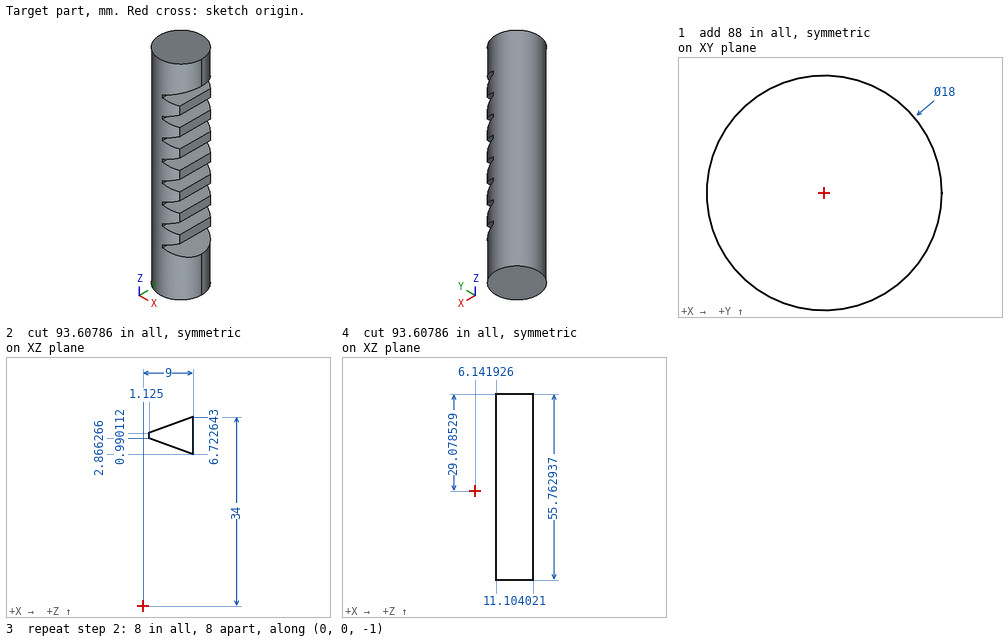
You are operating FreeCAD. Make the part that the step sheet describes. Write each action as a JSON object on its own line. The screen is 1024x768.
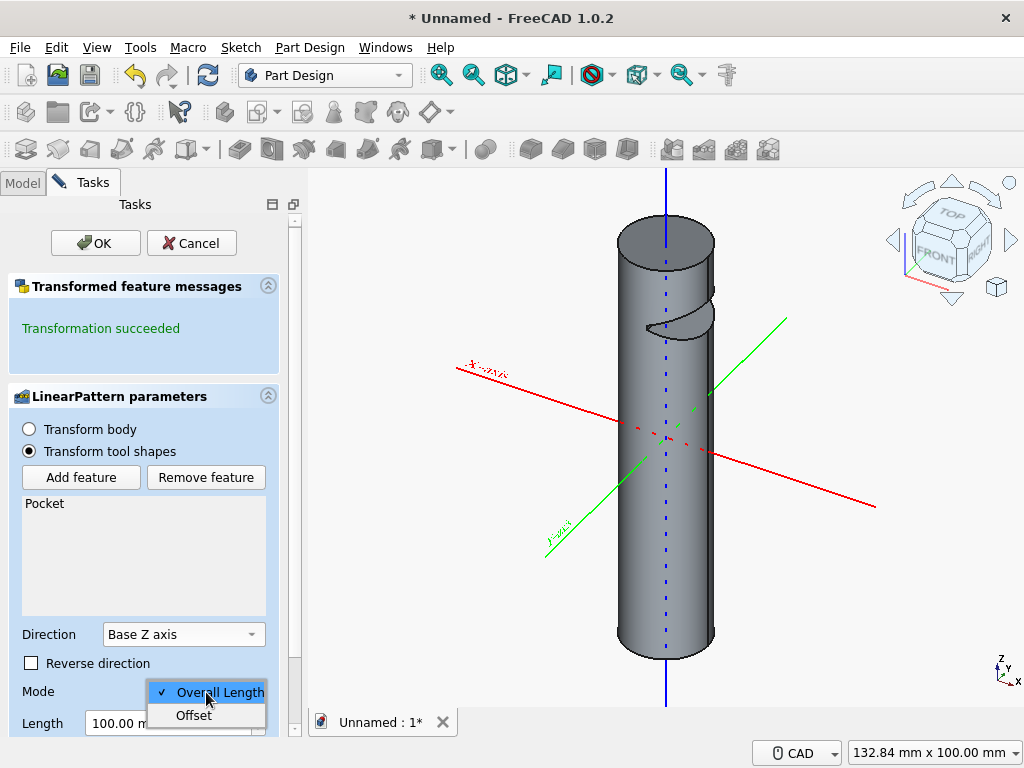
{"action": "left_click", "coordinate": [206, 716]}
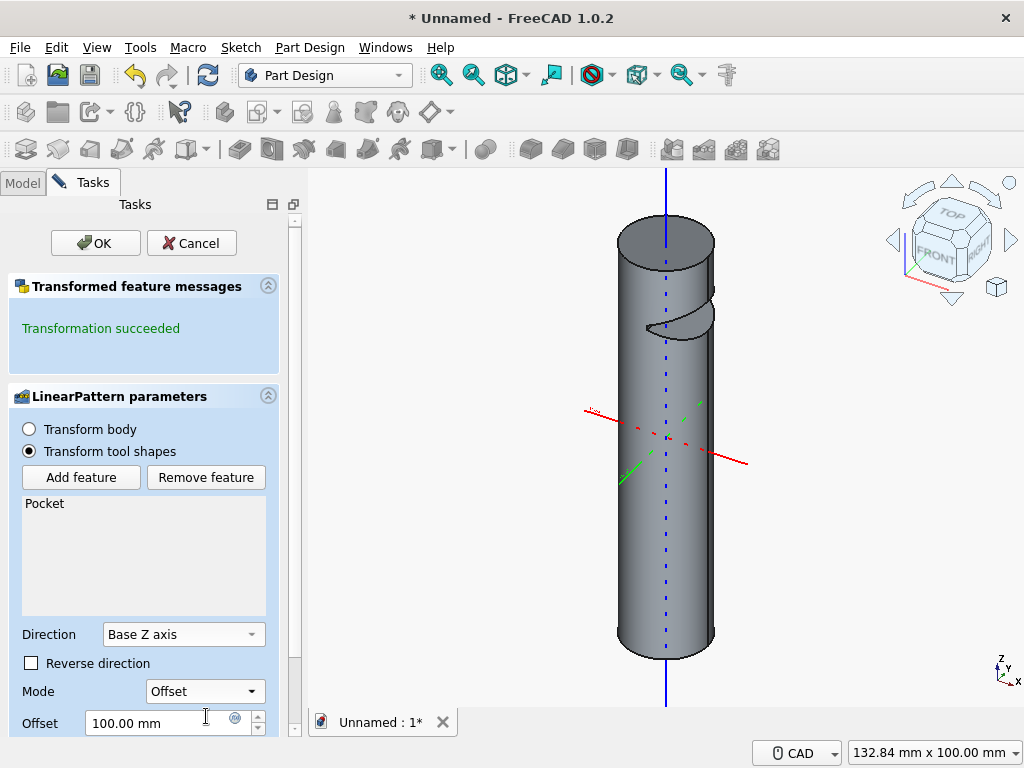
{"action": "triple_click", "coordinate": [168, 723]}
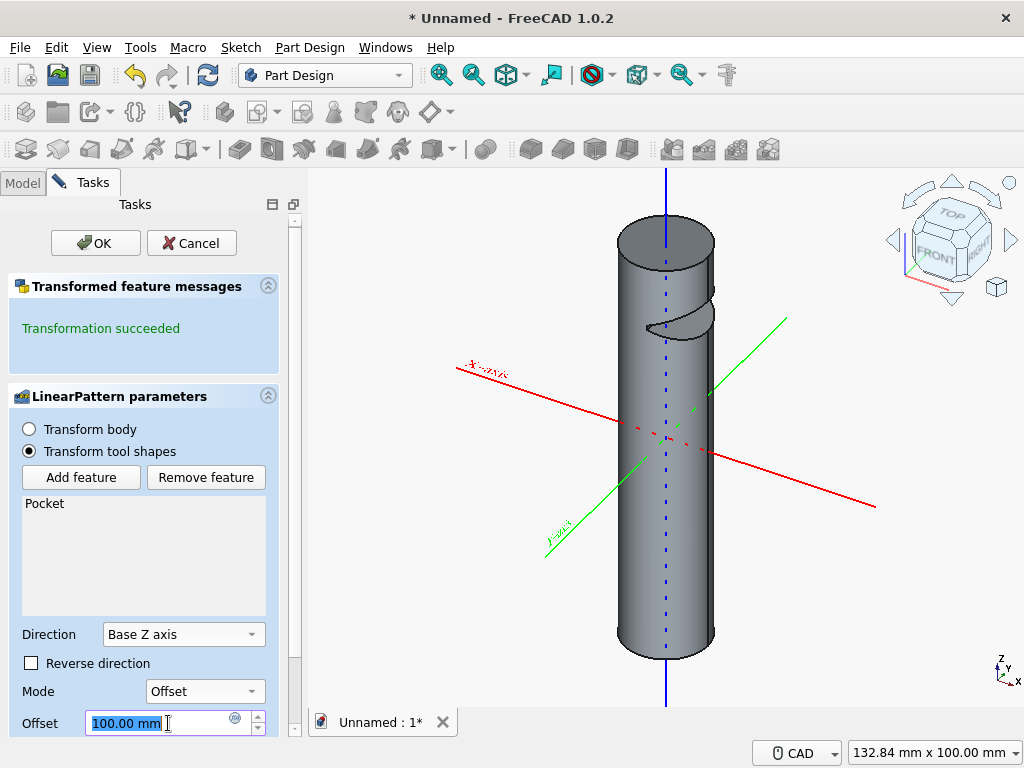
{"action": "type", "text": "8"}
{"action": "key", "text": "Tab"}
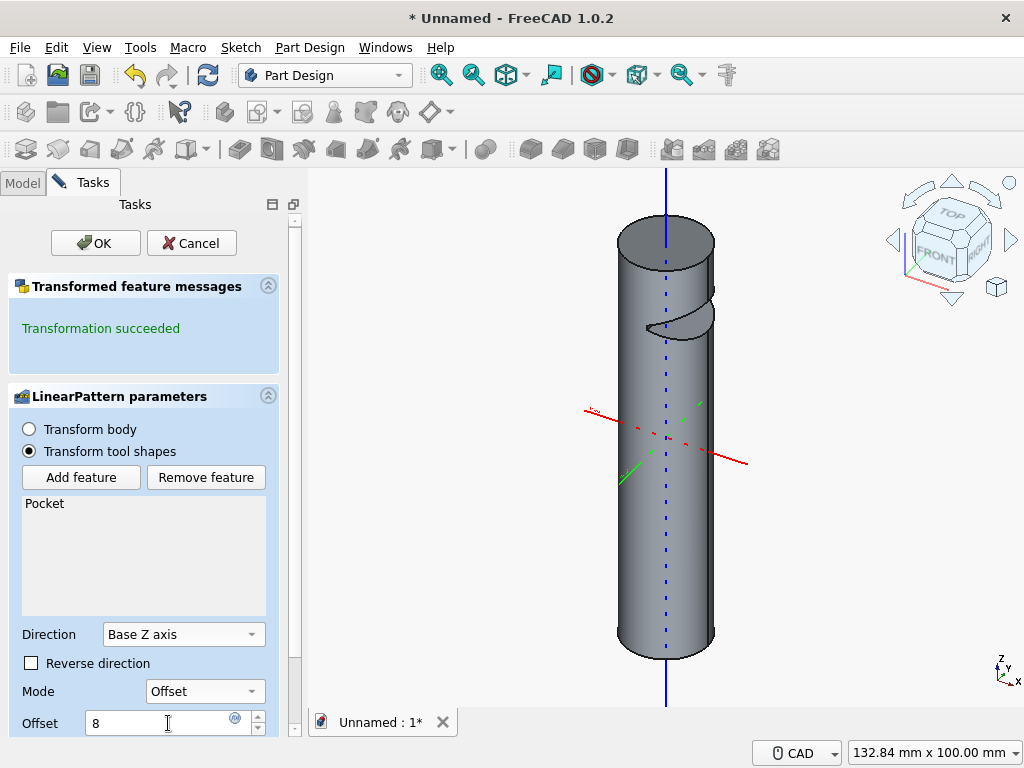
{"action": "scroll", "coordinate": [295, 475], "scroll_direction": "down", "scroll_amount": 2}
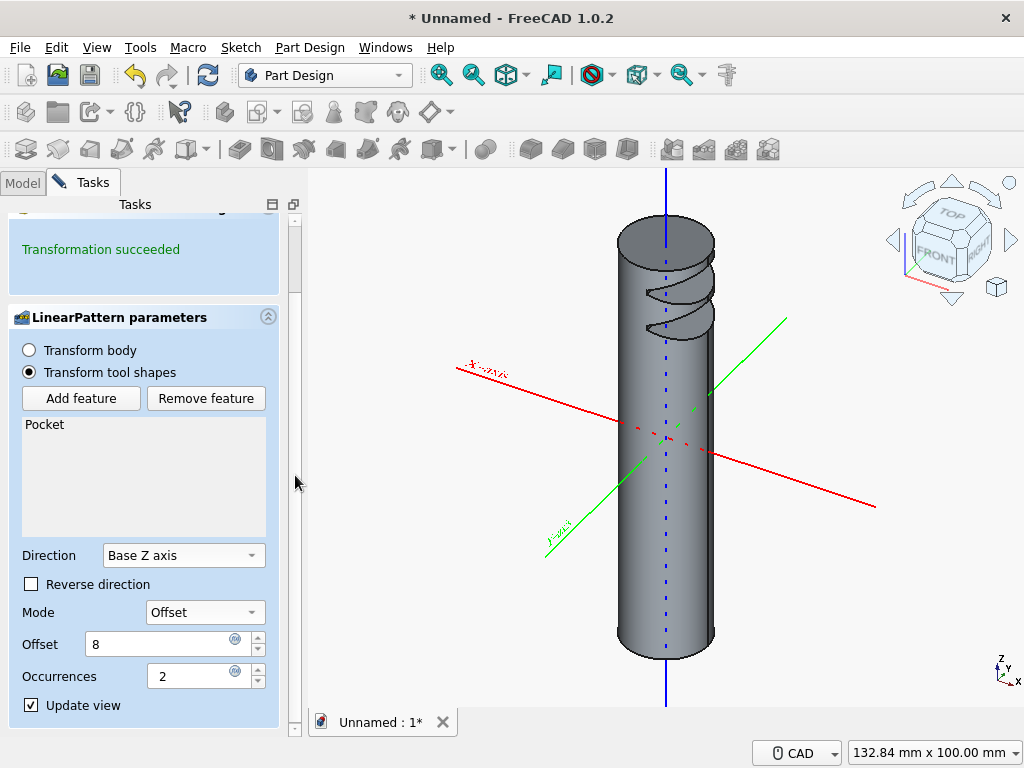
{"action": "triple_click", "coordinate": [198, 676]}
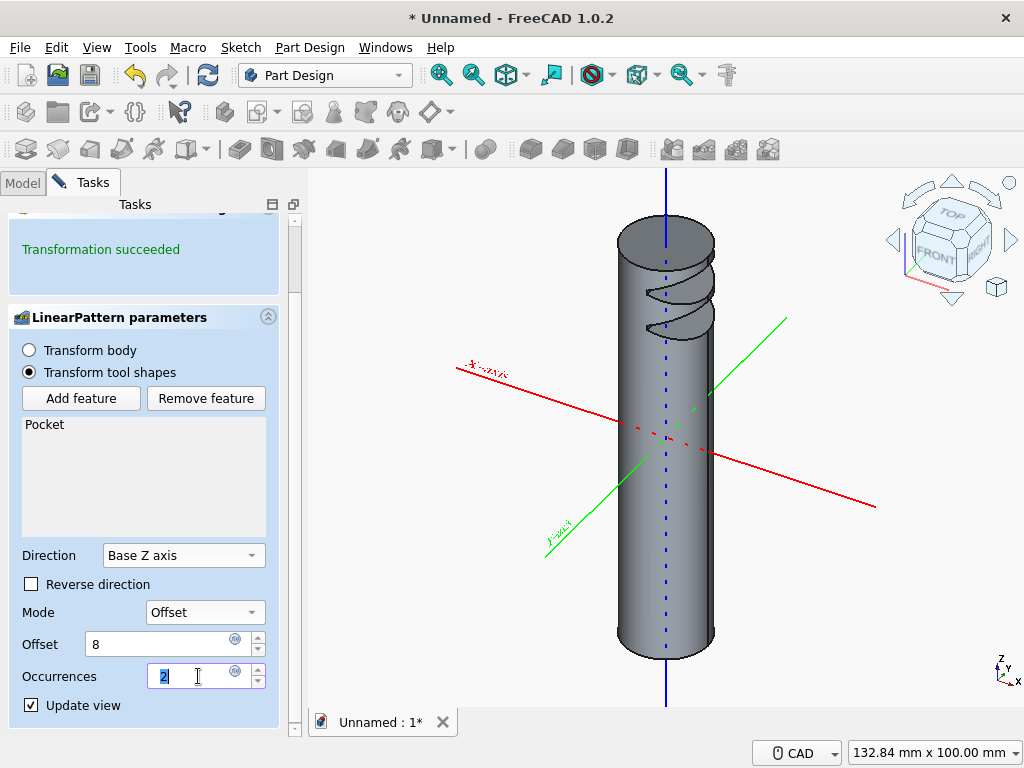
{"action": "type", "text": "8"}
{"action": "key", "text": "Tab"}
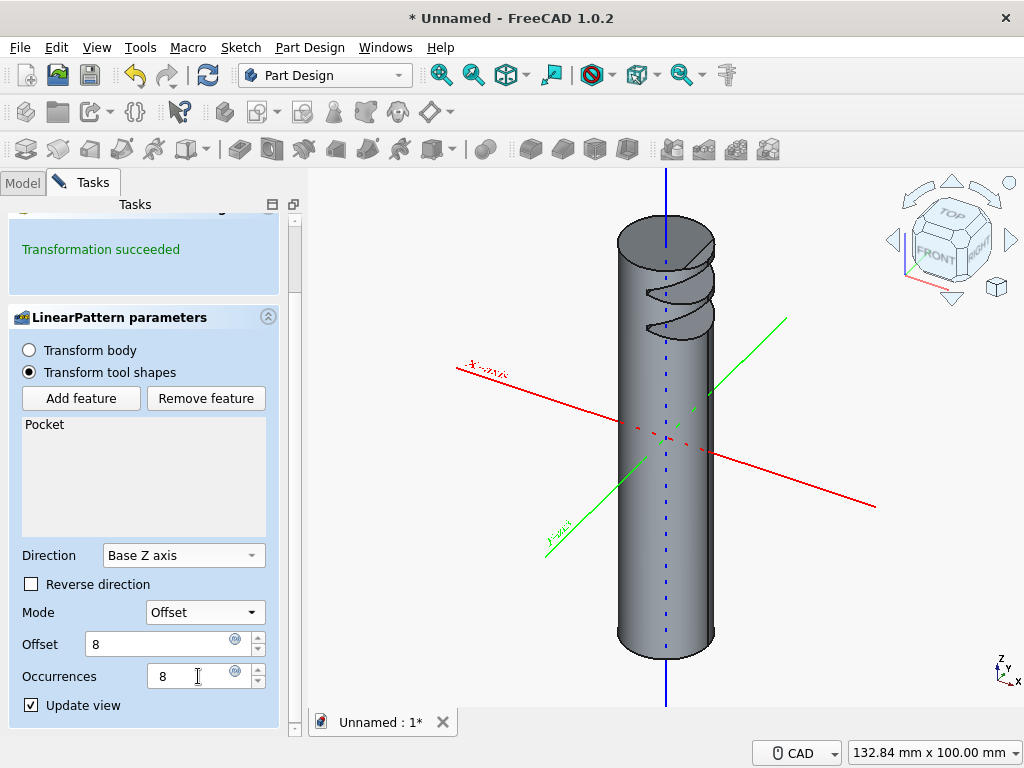
{"action": "left_click", "coordinate": [30, 584]}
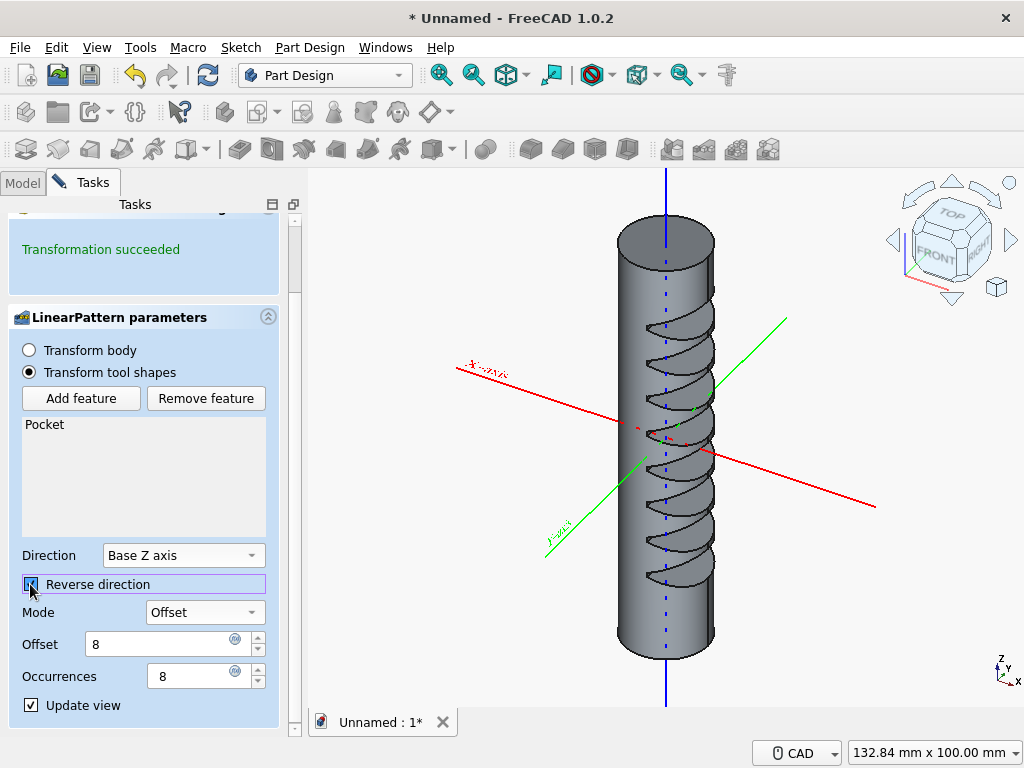
{"action": "scroll", "coordinate": [295, 475], "scroll_direction": "up", "scroll_amount": 3}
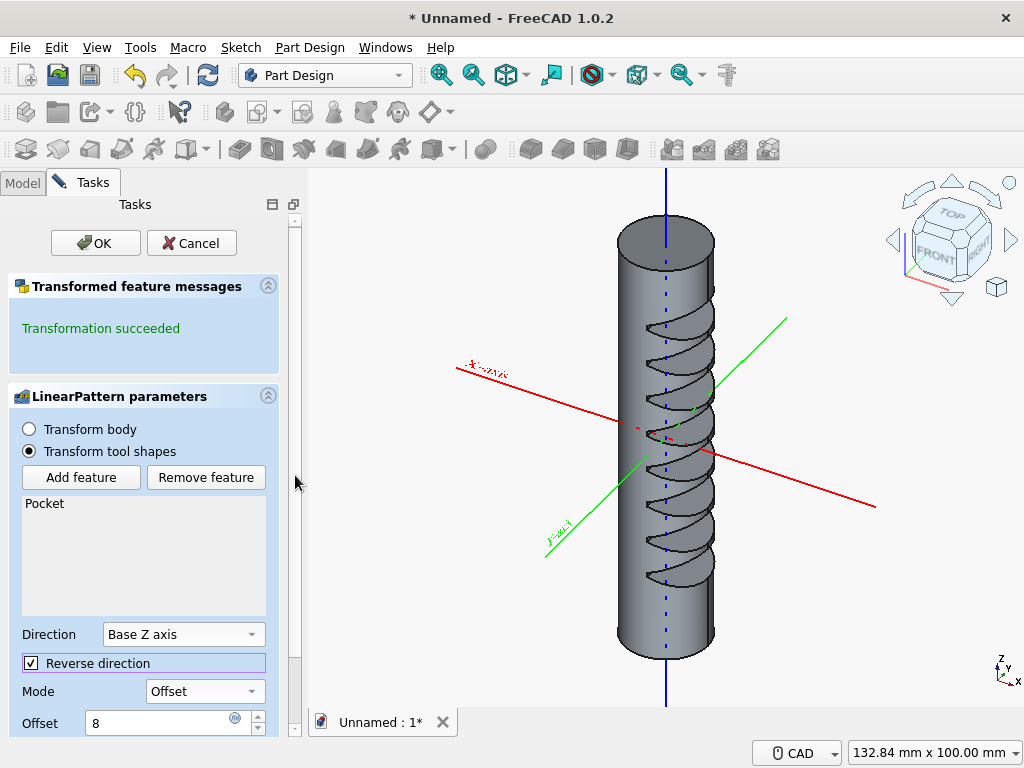
{"action": "left_click", "coordinate": [96, 243]}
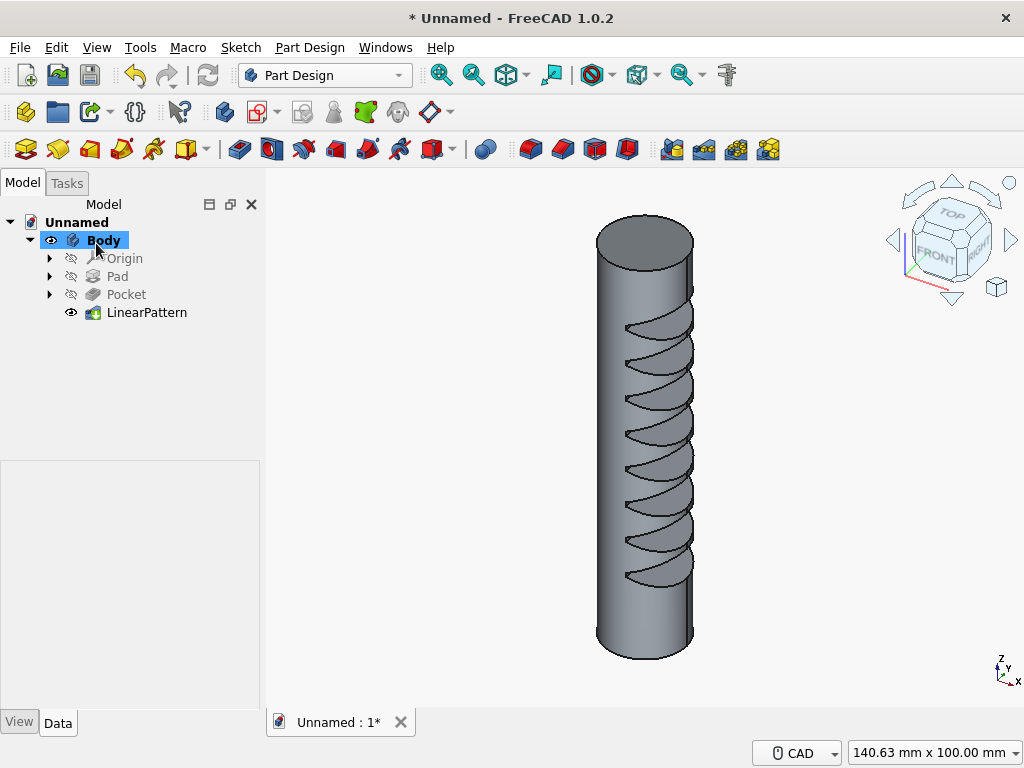
{"action": "left_click", "coordinate": [258, 112]}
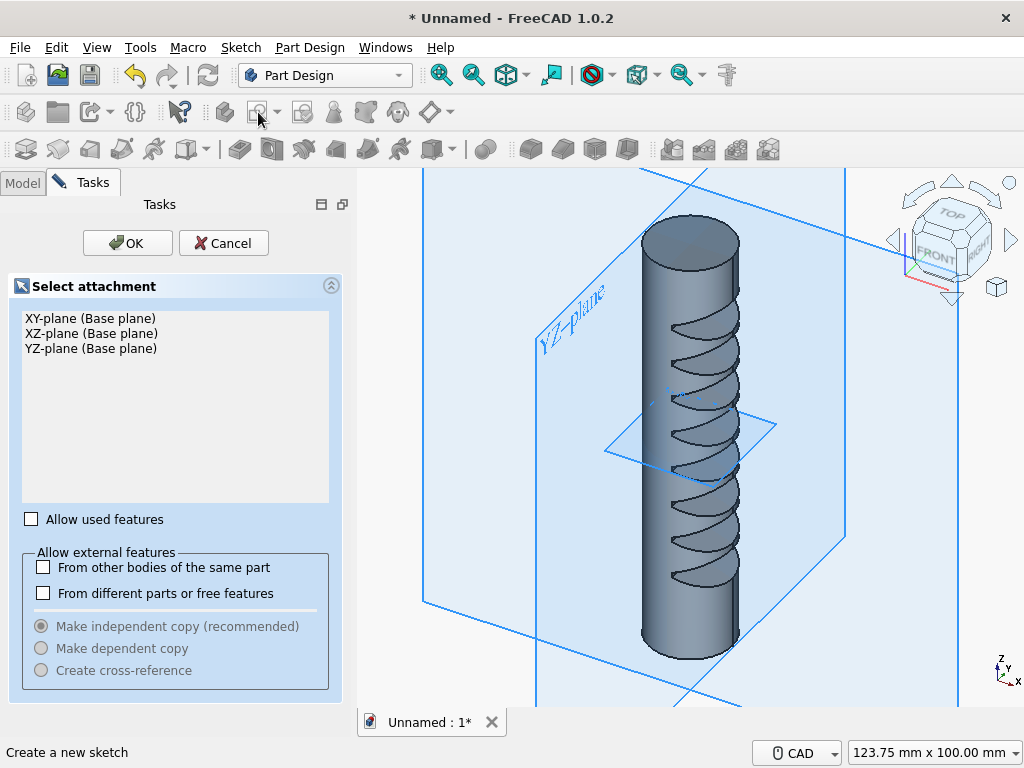
{"action": "left_click", "coordinate": [82, 334]}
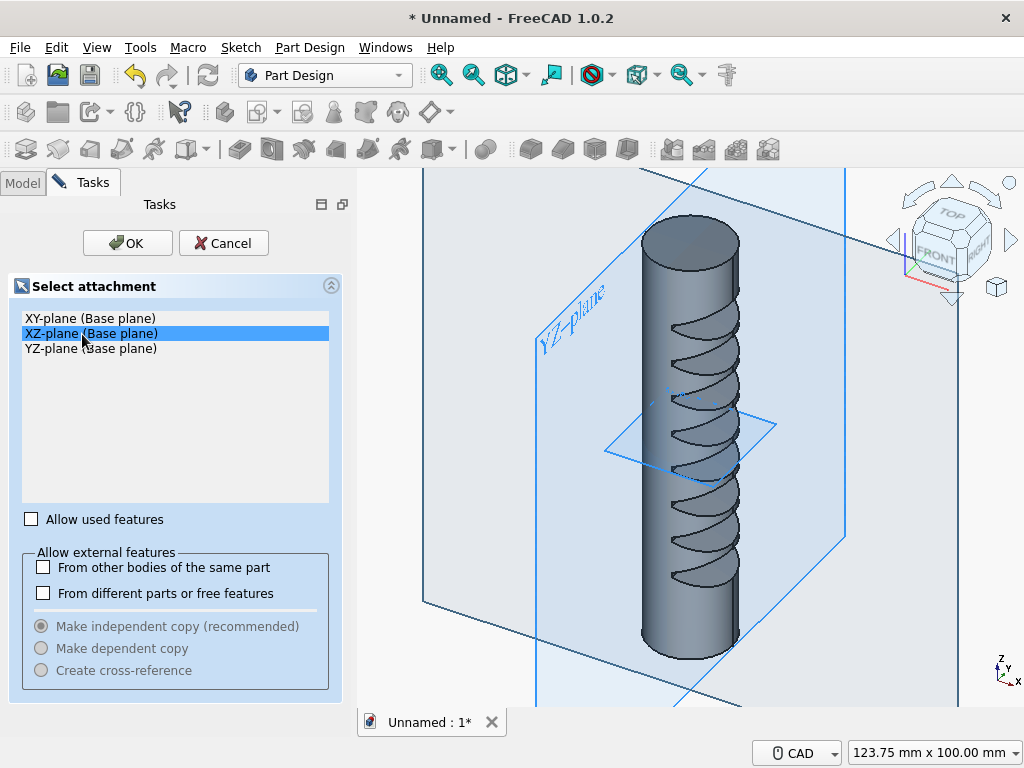
{"action": "left_click", "coordinate": [128, 243]}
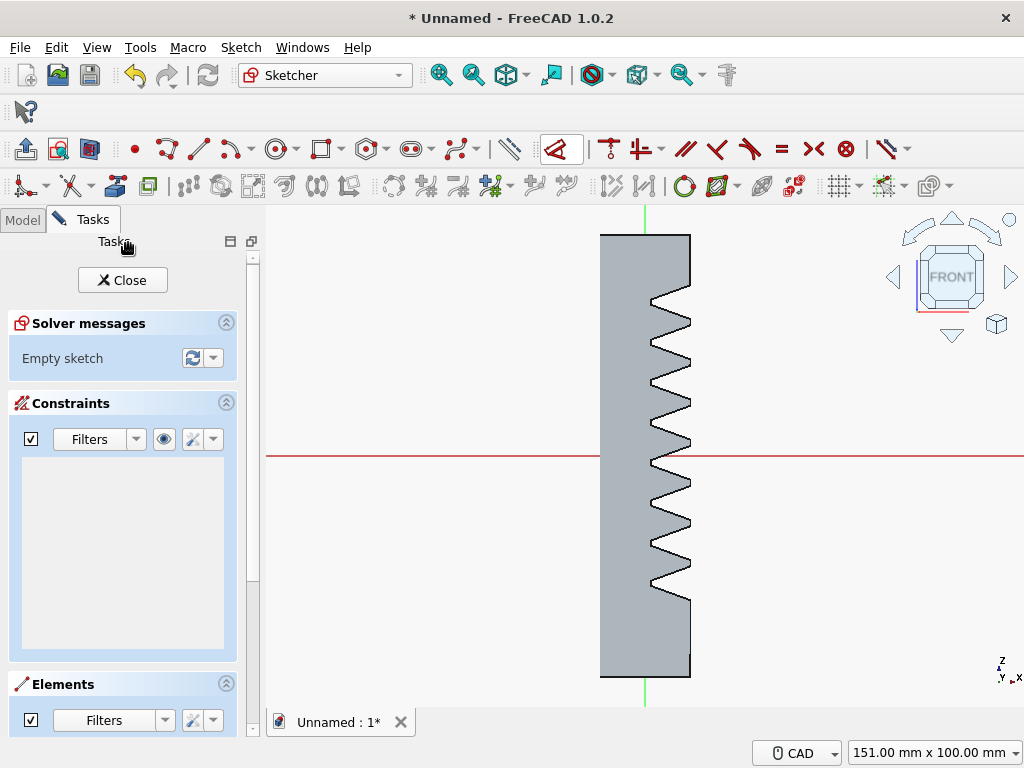
{"action": "left_click", "coordinate": [90, 150]}